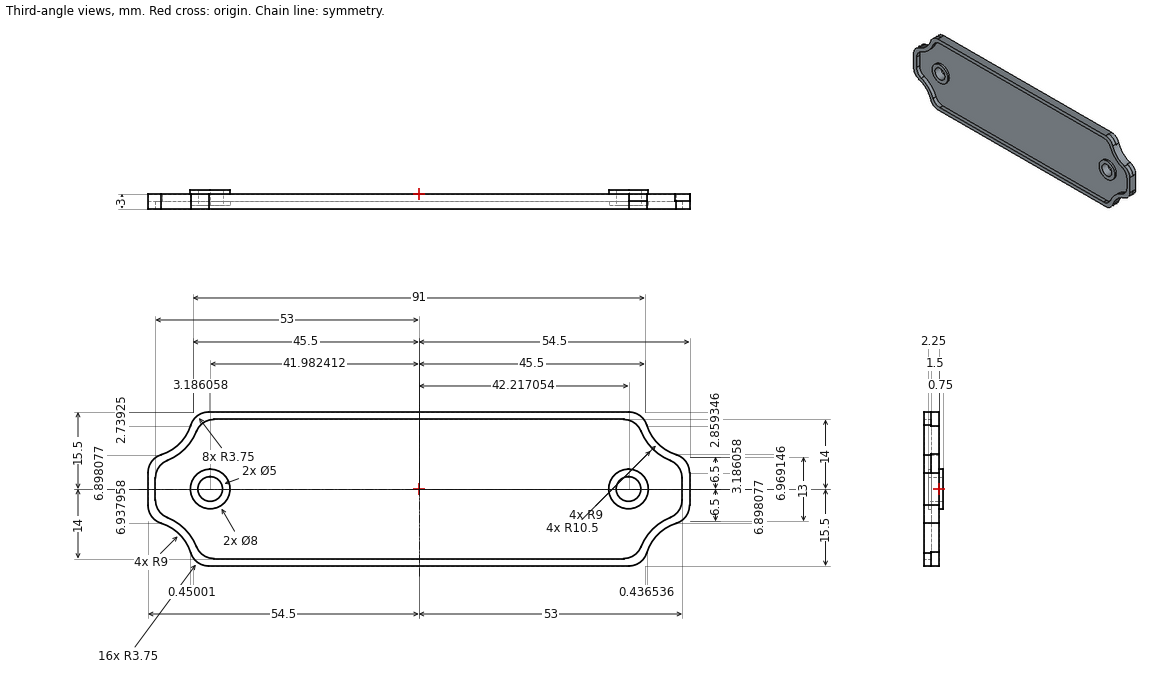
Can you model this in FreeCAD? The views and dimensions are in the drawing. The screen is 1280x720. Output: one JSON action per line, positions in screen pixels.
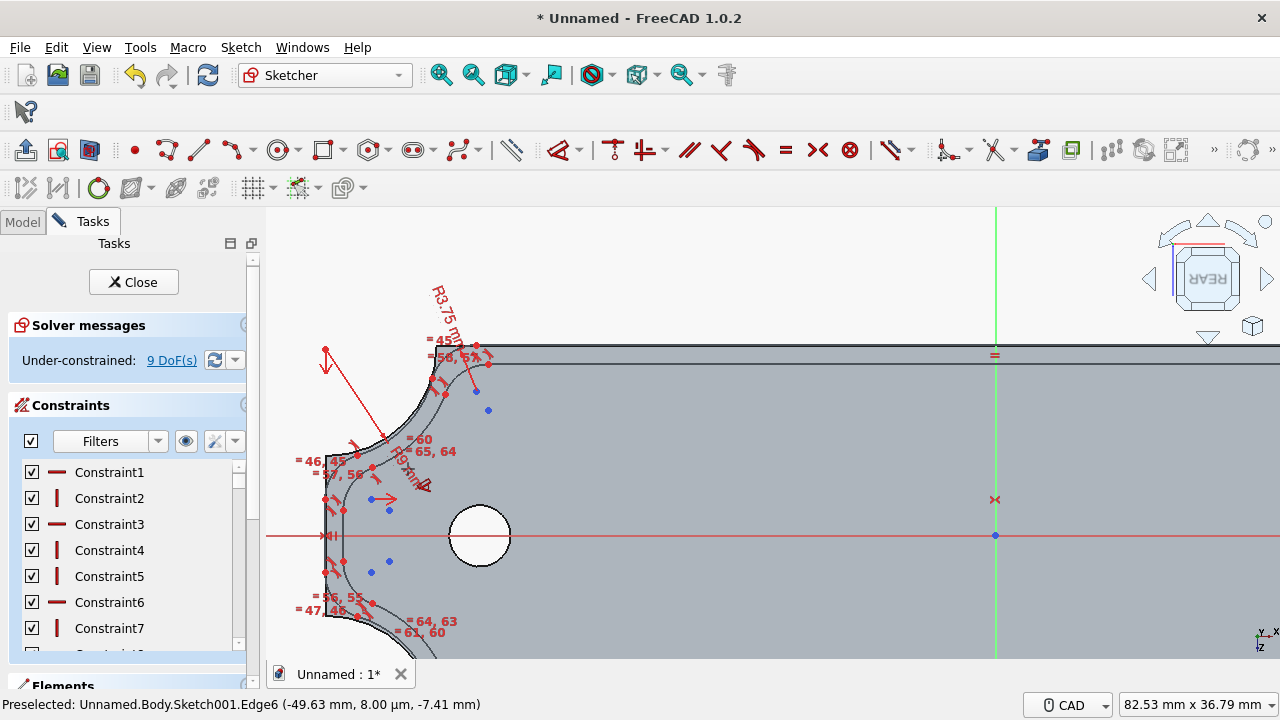
{"action": "scroll", "coordinate": [467, 349], "scroll_direction": "down", "scroll_amount": 4}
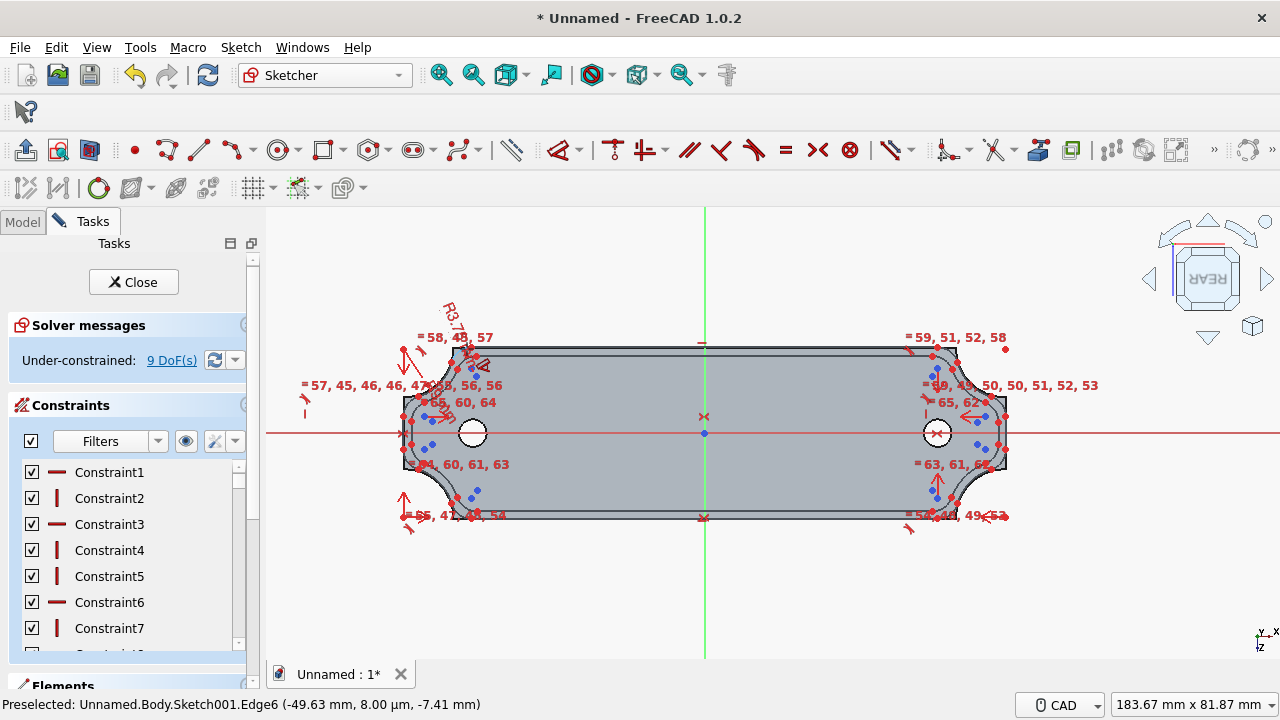
{"action": "scroll", "coordinate": [972, 471], "scroll_direction": "up", "scroll_amount": 4}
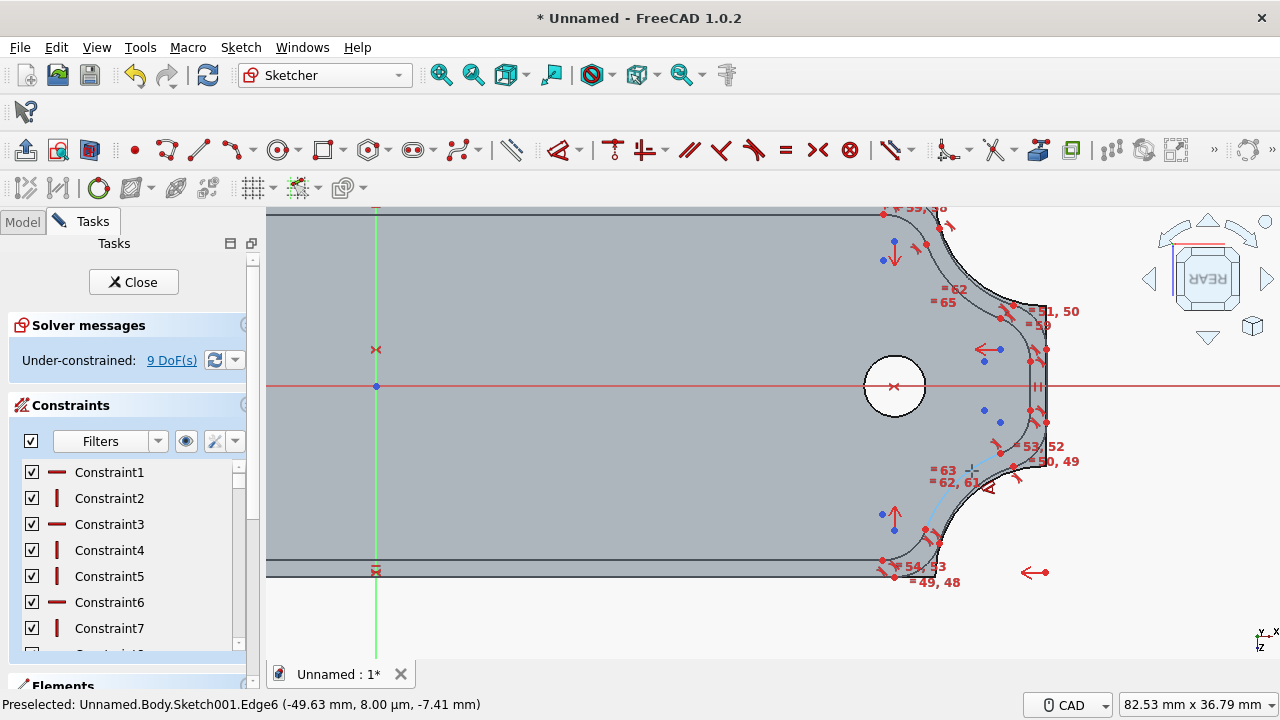
{"action": "left_click", "coordinate": [972, 469]}
{"action": "left_click", "coordinate": [953, 443]}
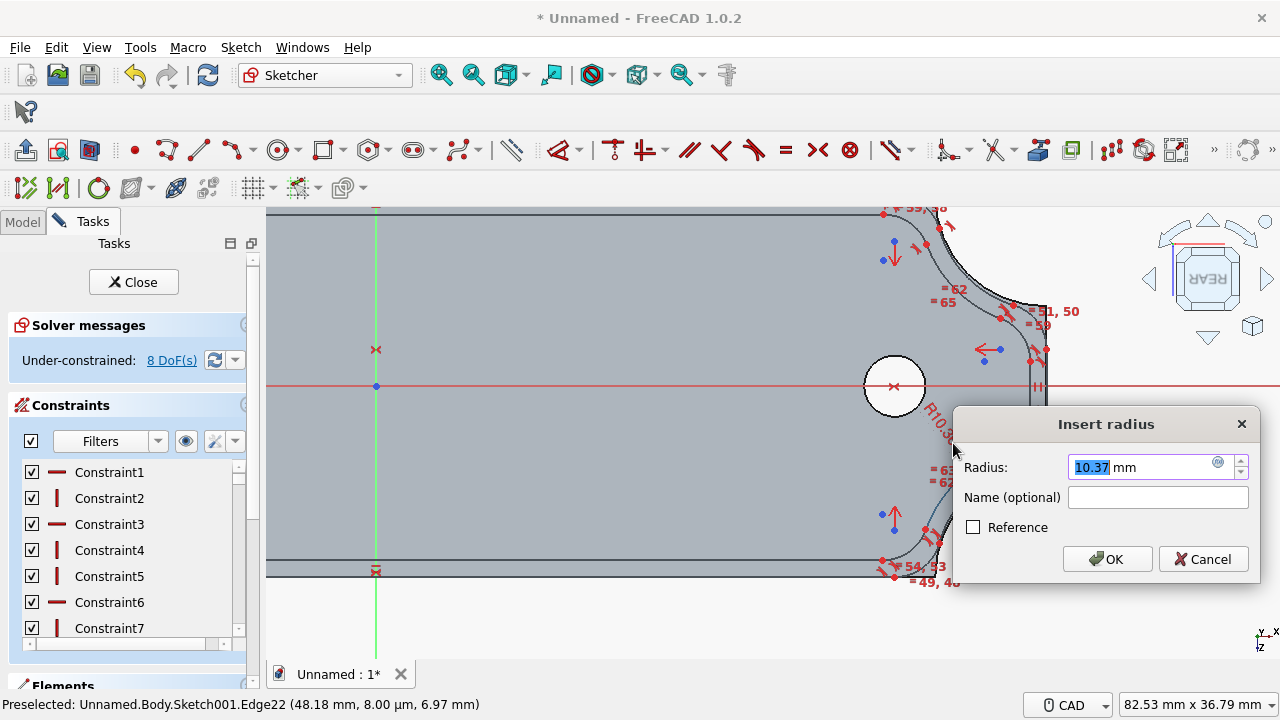
{"action": "type", "text": "10.5"}
{"action": "key", "text": "Return"}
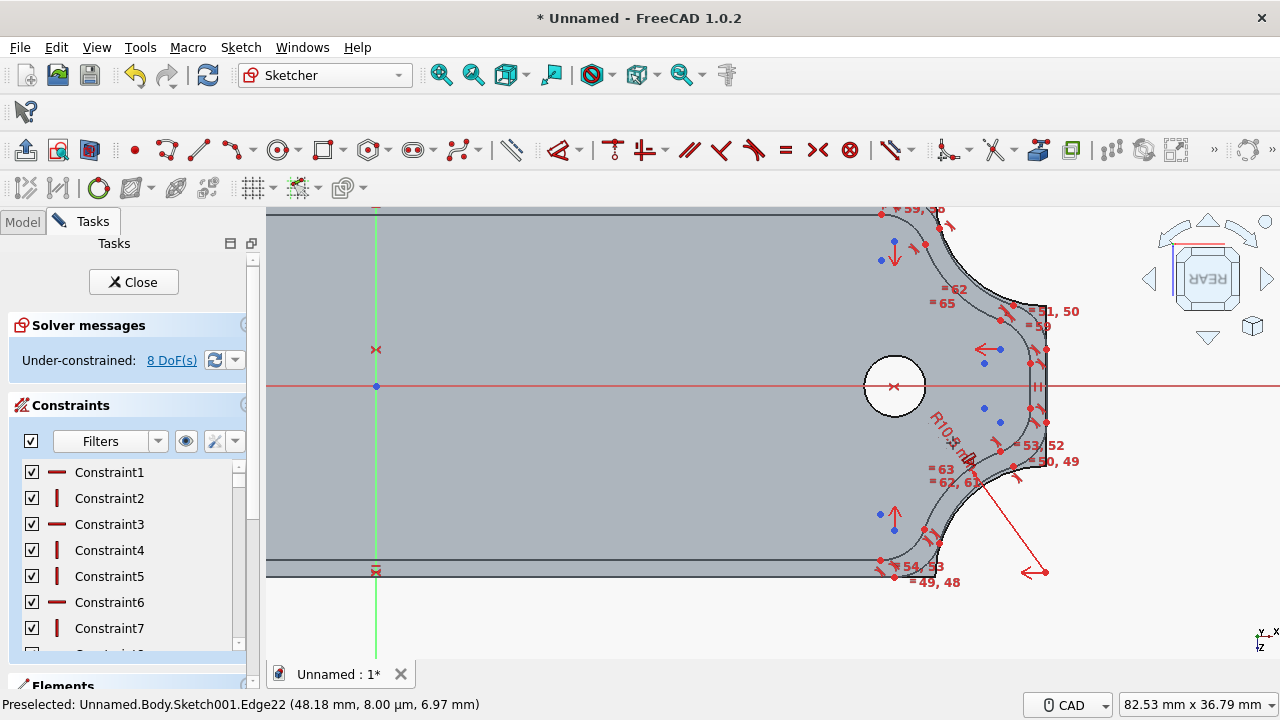
{"action": "left_click", "coordinate": [1030, 363]}
{"action": "left_click", "coordinate": [703, 329]}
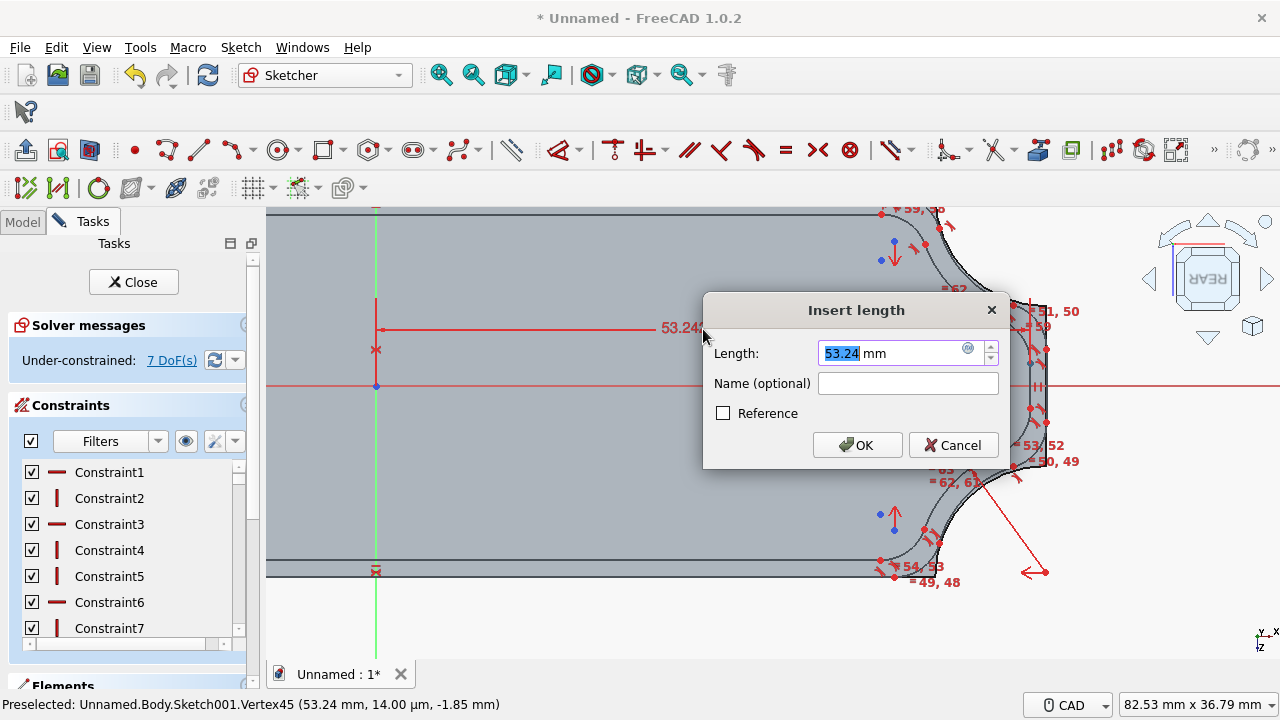
{"action": "type", "text": "53"}
{"action": "key", "text": "Return"}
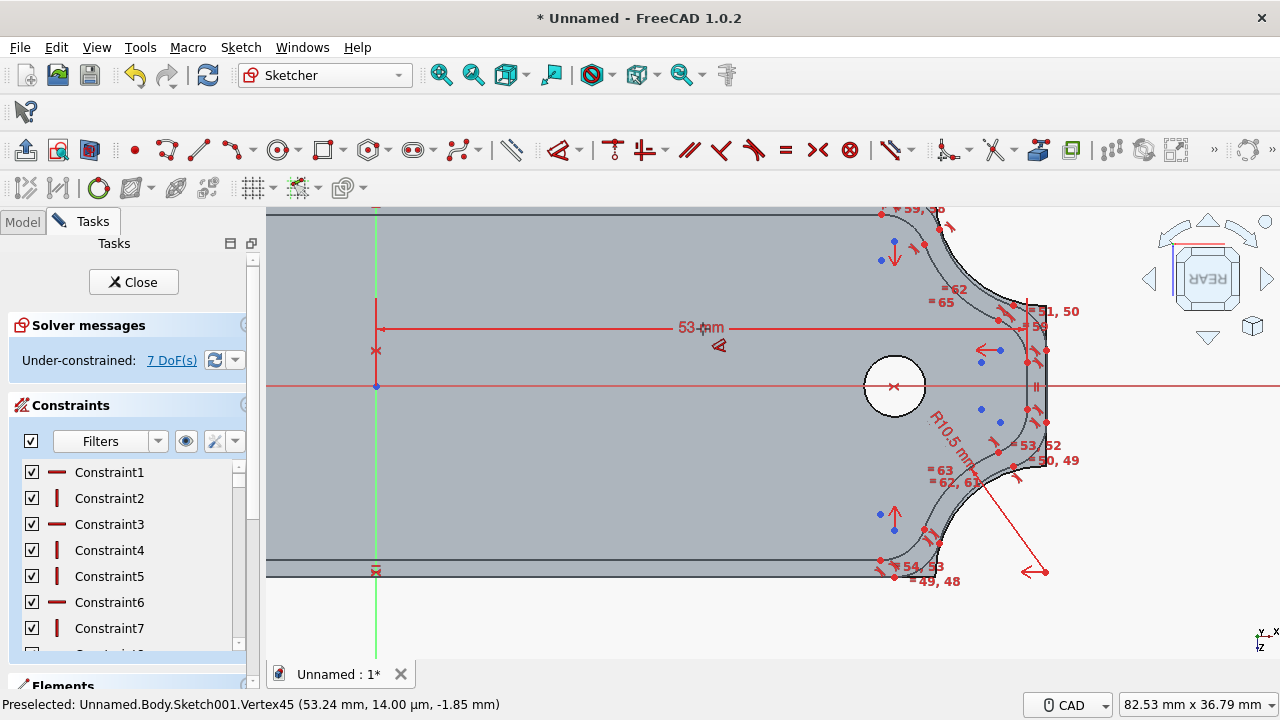
{"action": "left_click", "coordinate": [881, 560]}
{"action": "left_click", "coordinate": [915, 473]}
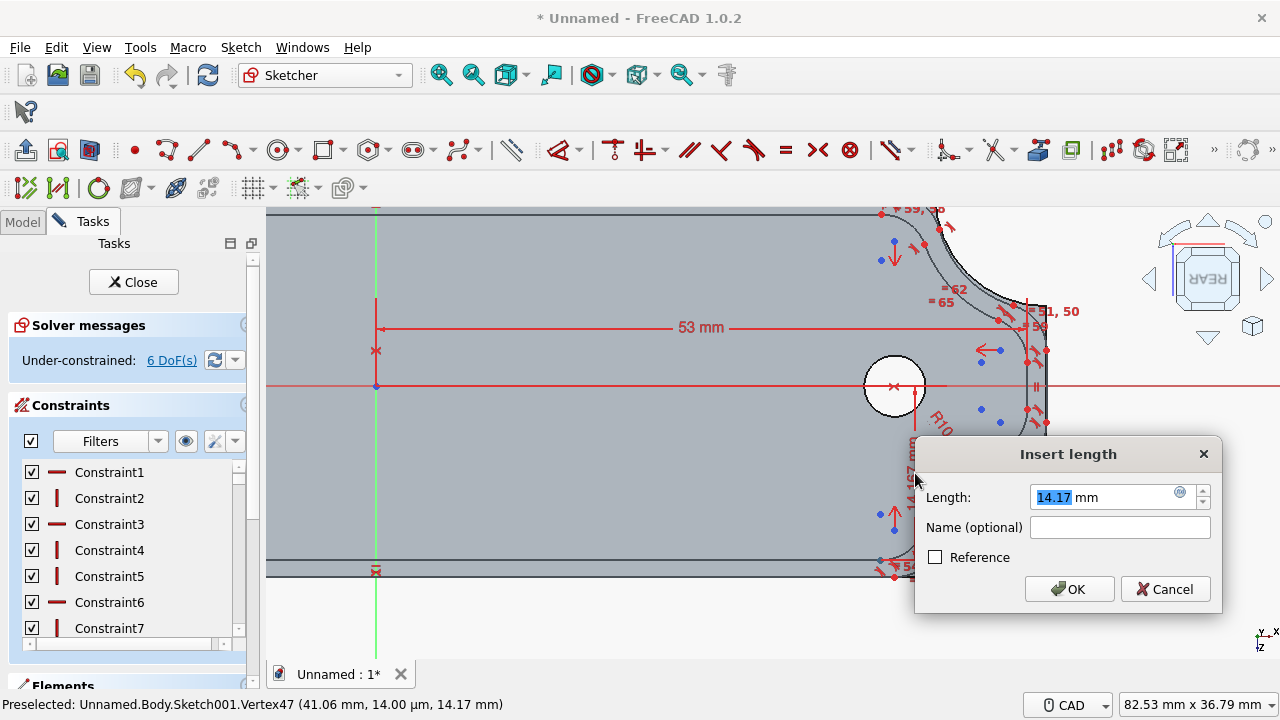
{"action": "type", "text": "14"}
{"action": "key", "text": "Return"}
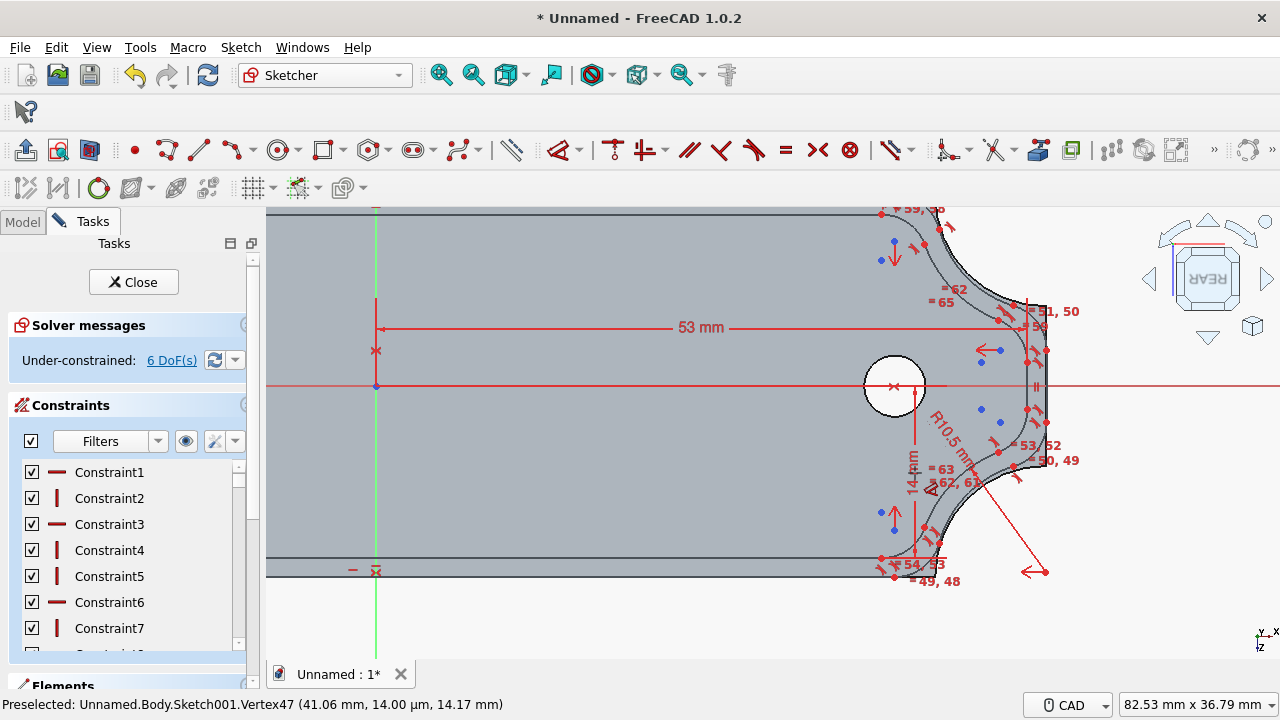
{"action": "scroll", "coordinate": [972, 471], "scroll_direction": "down", "scroll_amount": 4}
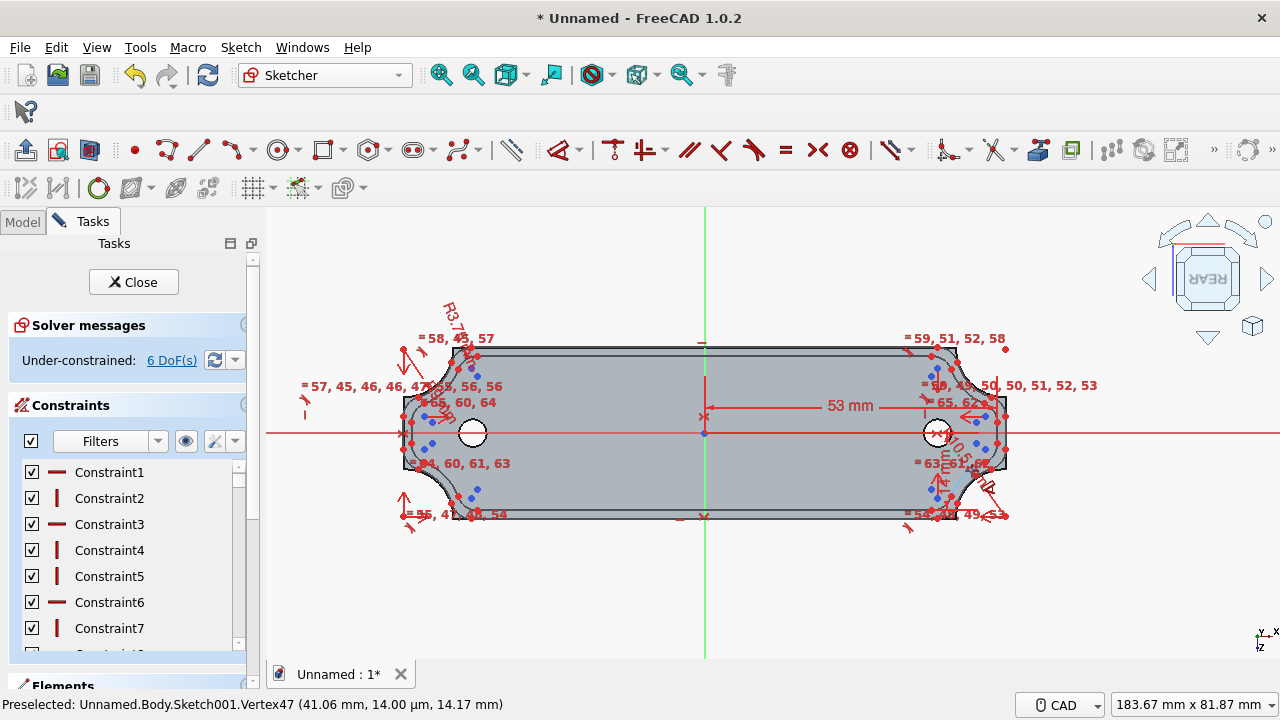
{"action": "left_click", "coordinate": [412, 443]}
{"action": "left_click", "coordinate": [558, 477]}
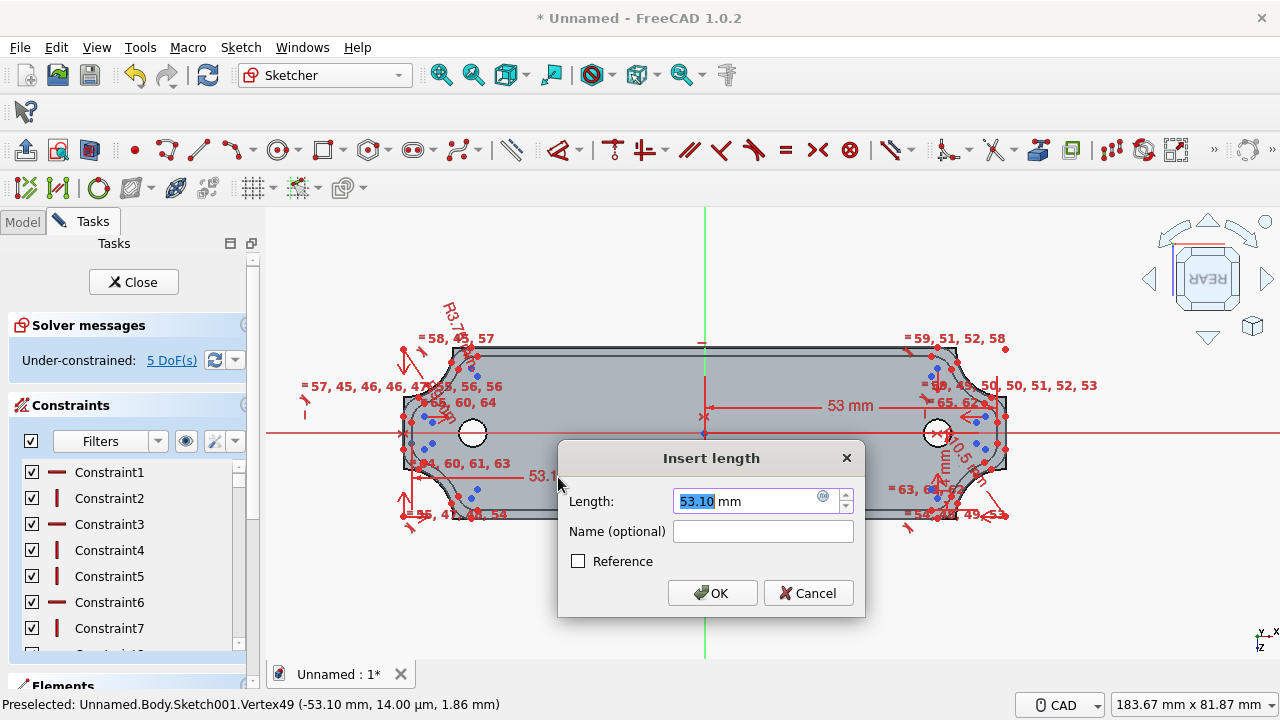
{"action": "type", "text": "53"}
{"action": "key", "text": "Return"}